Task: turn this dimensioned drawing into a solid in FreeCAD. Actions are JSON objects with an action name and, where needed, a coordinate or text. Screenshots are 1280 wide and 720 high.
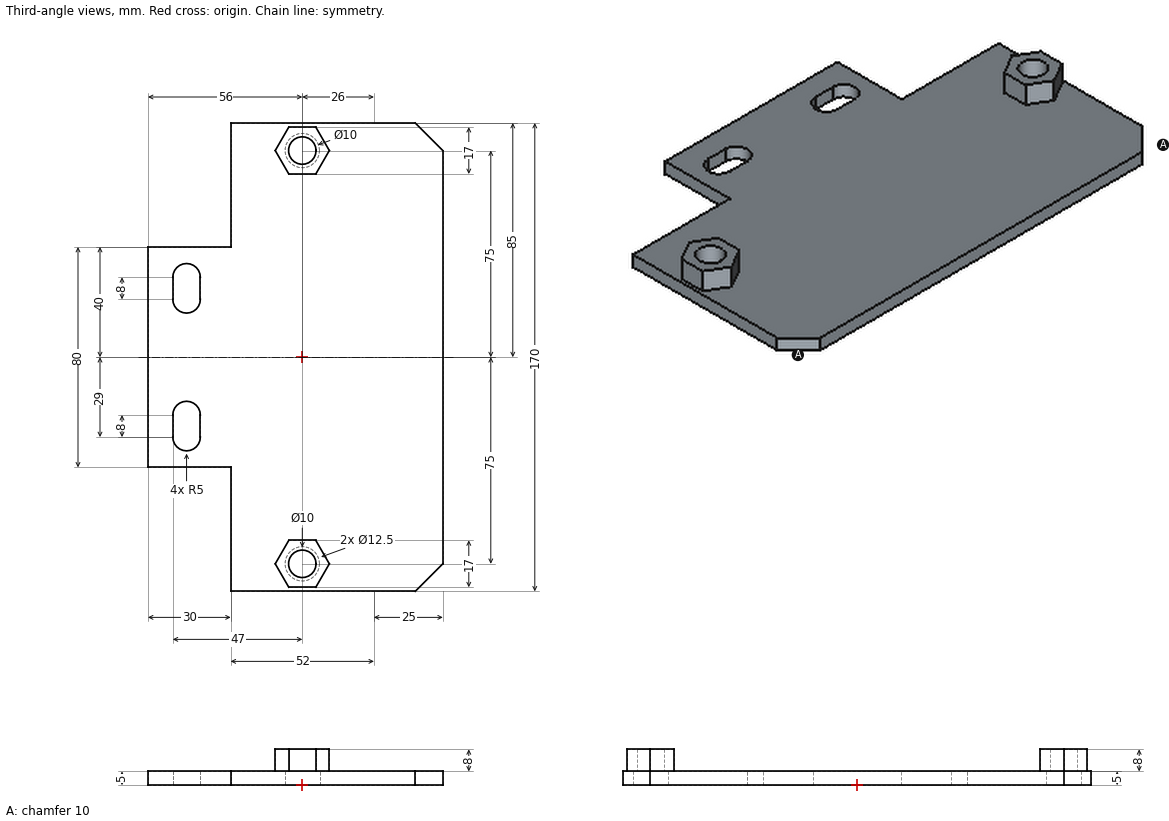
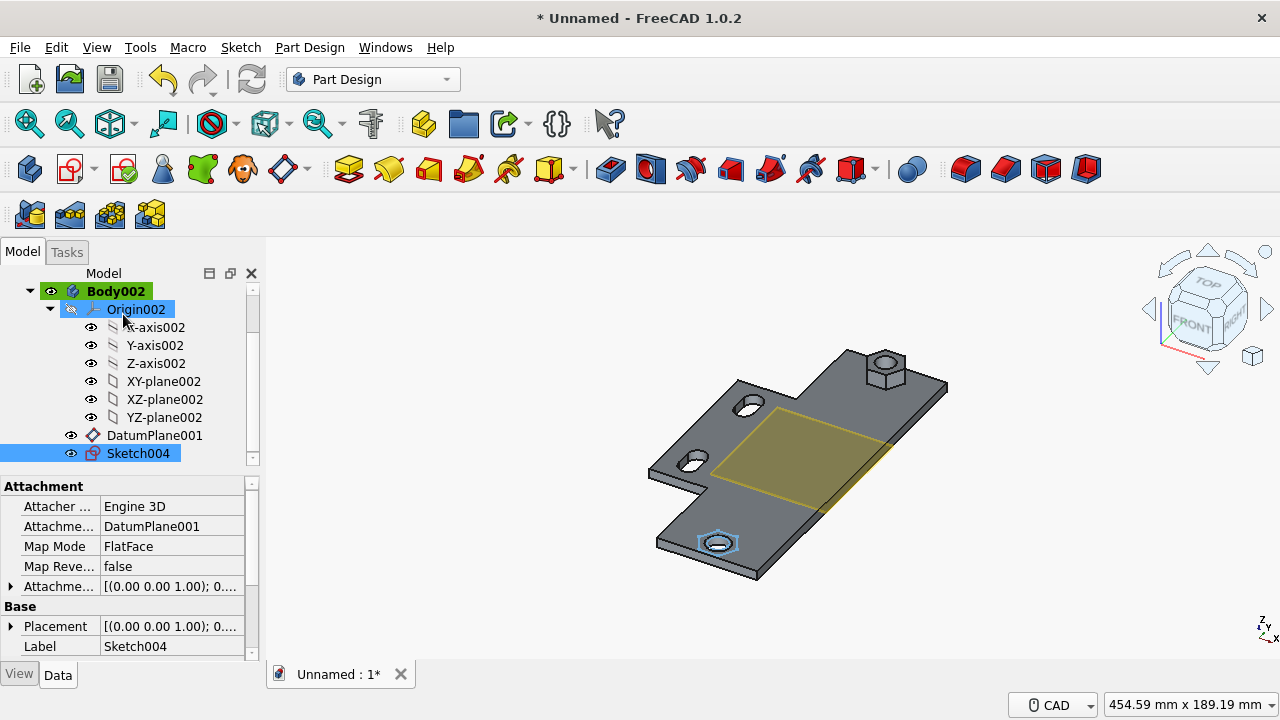
{"action": "left_click", "coordinate": [350, 170]}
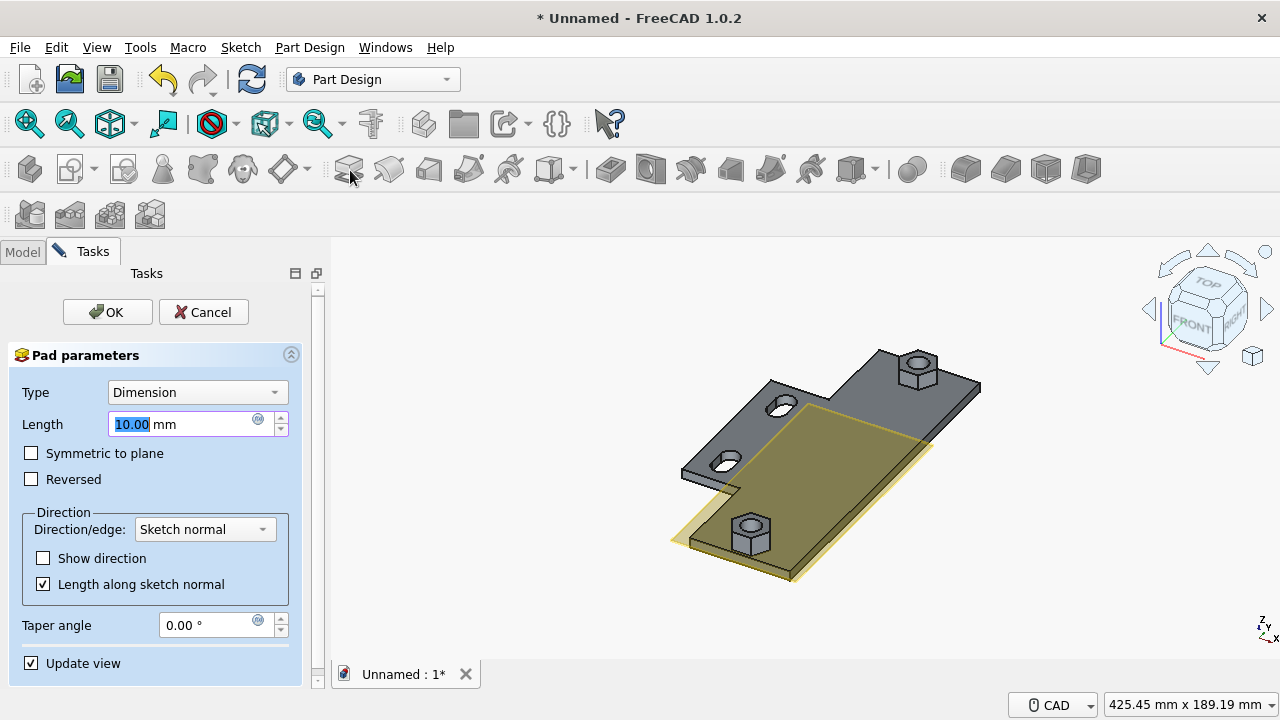
{"action": "type", "text": "8"}
{"action": "key", "text": "Tab"}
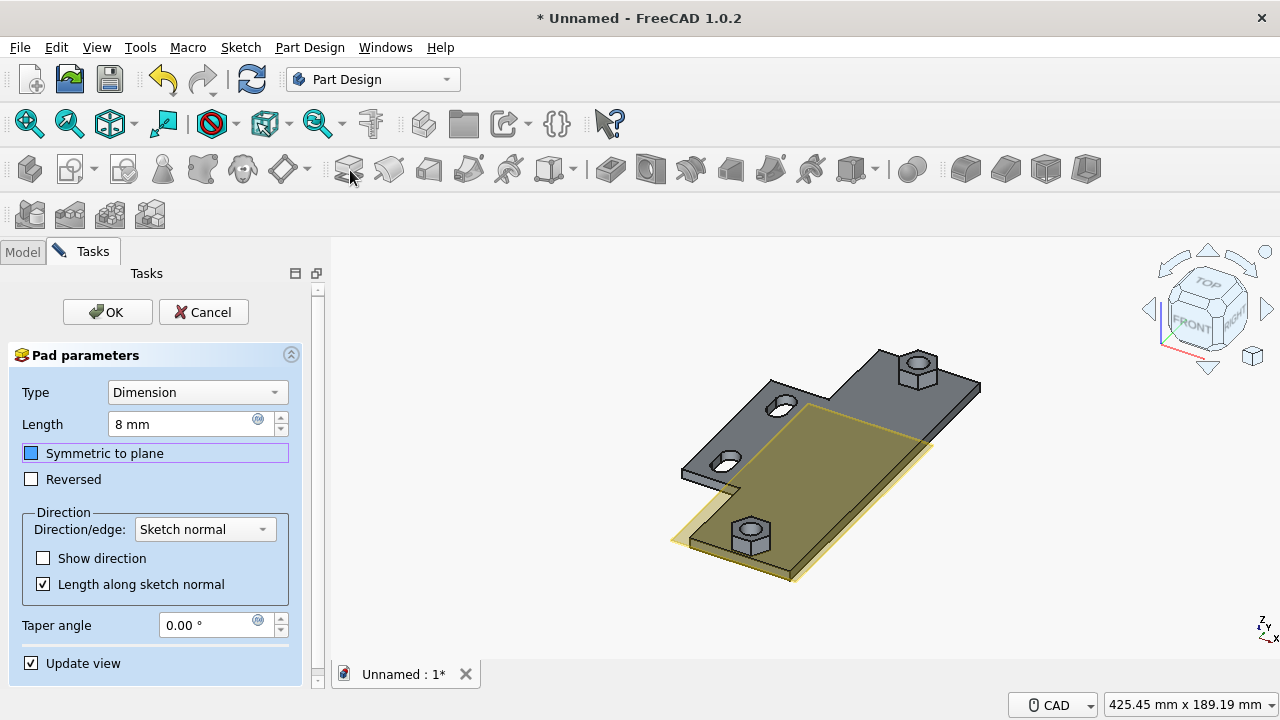
{"action": "left_click", "coordinate": [108, 312]}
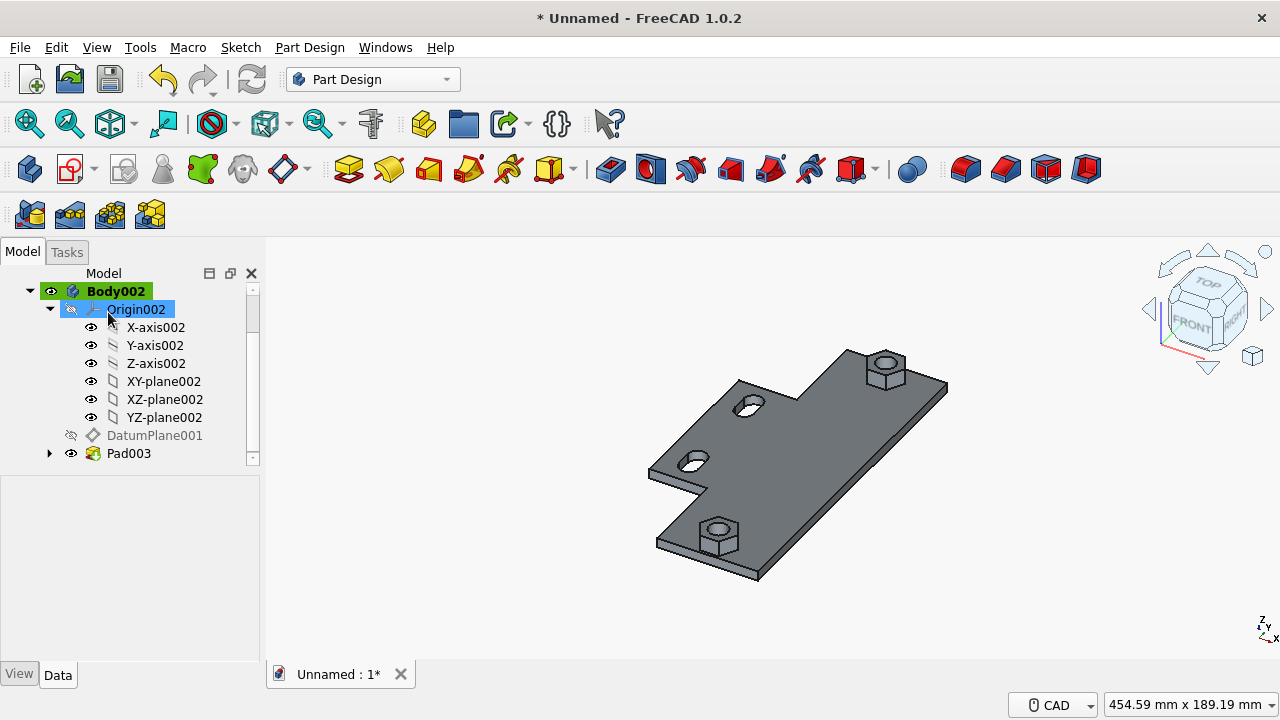
{"action": "left_click", "coordinate": [30, 124]}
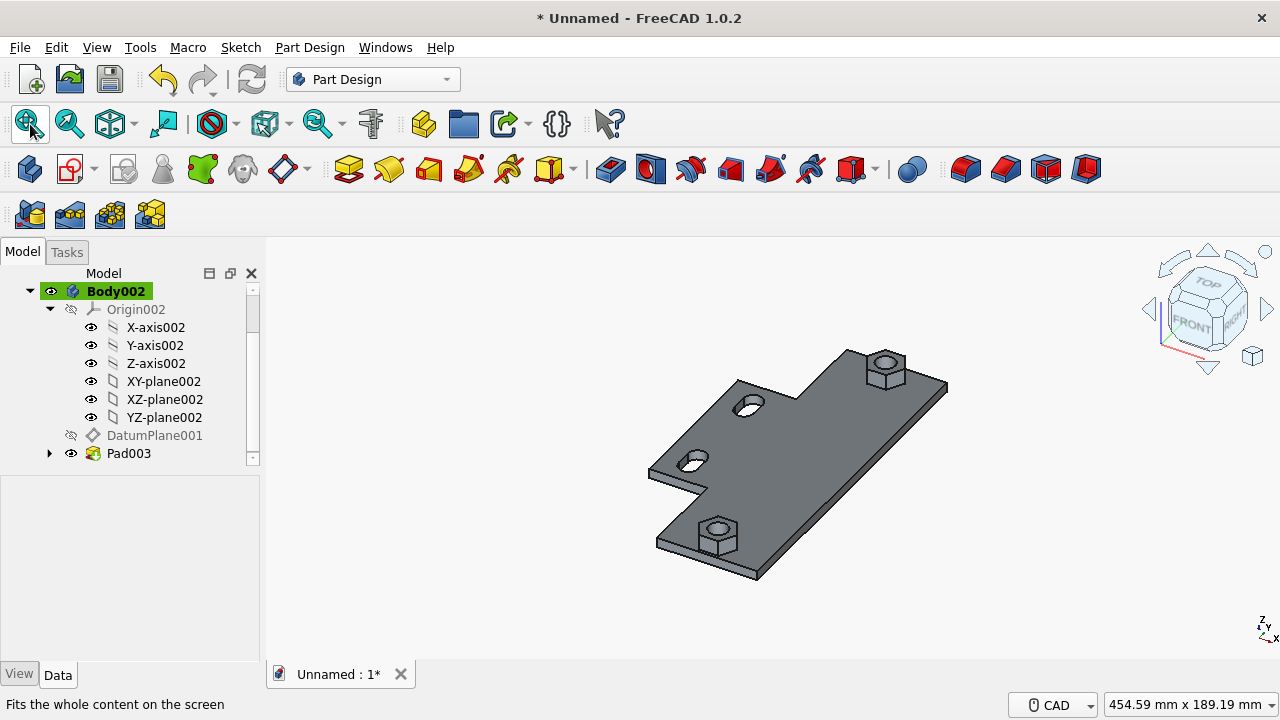
{"action": "left_click", "coordinate": [30, 170]}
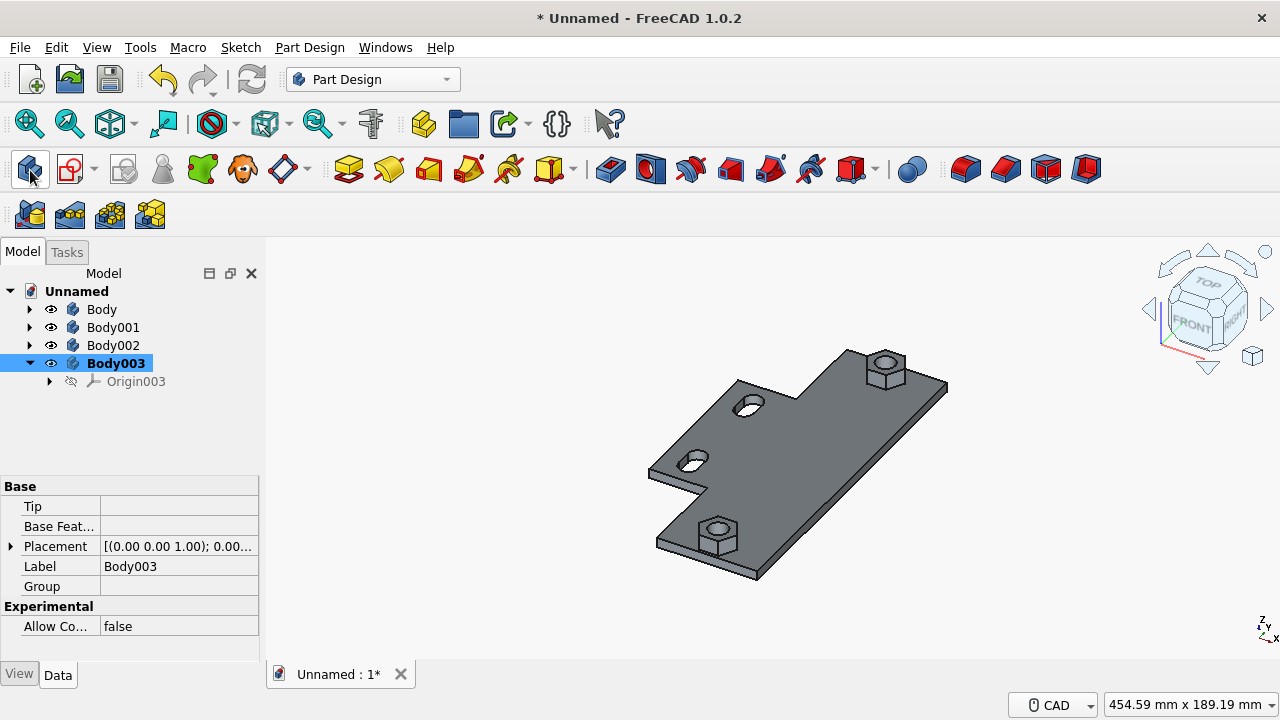
{"action": "left_click", "coordinate": [50, 381]}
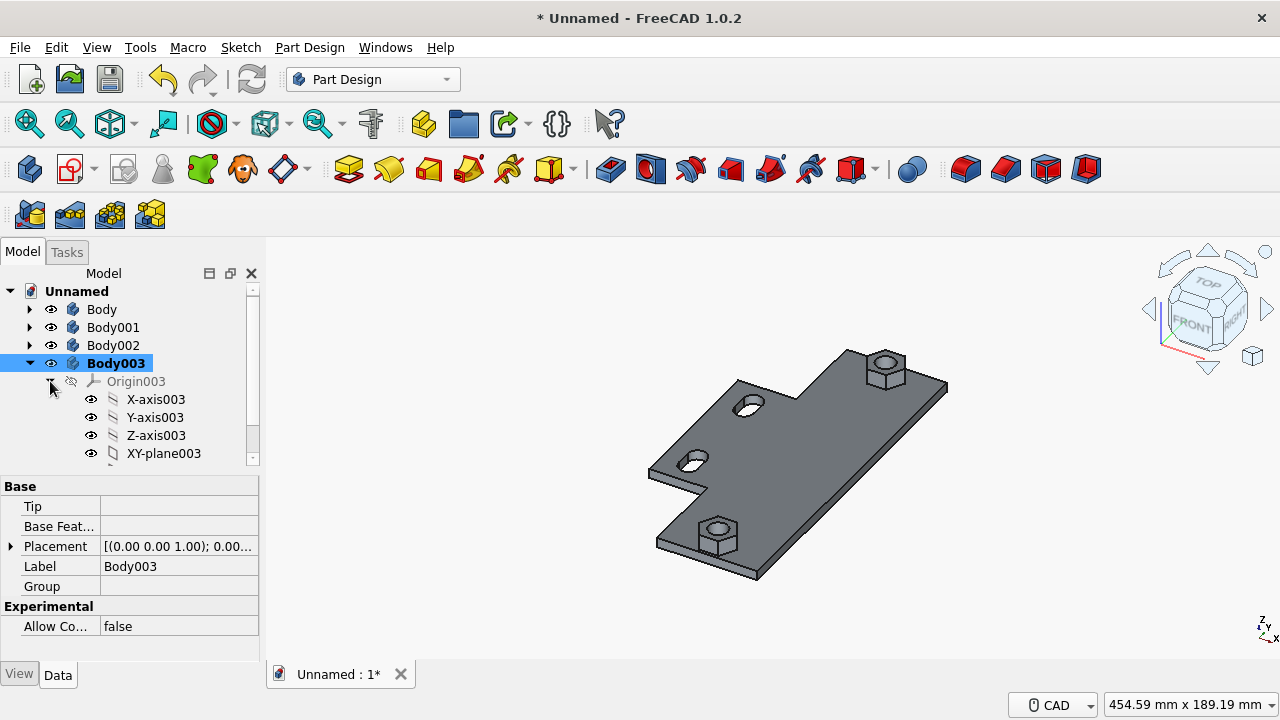
{"action": "left_click", "coordinate": [136, 453]}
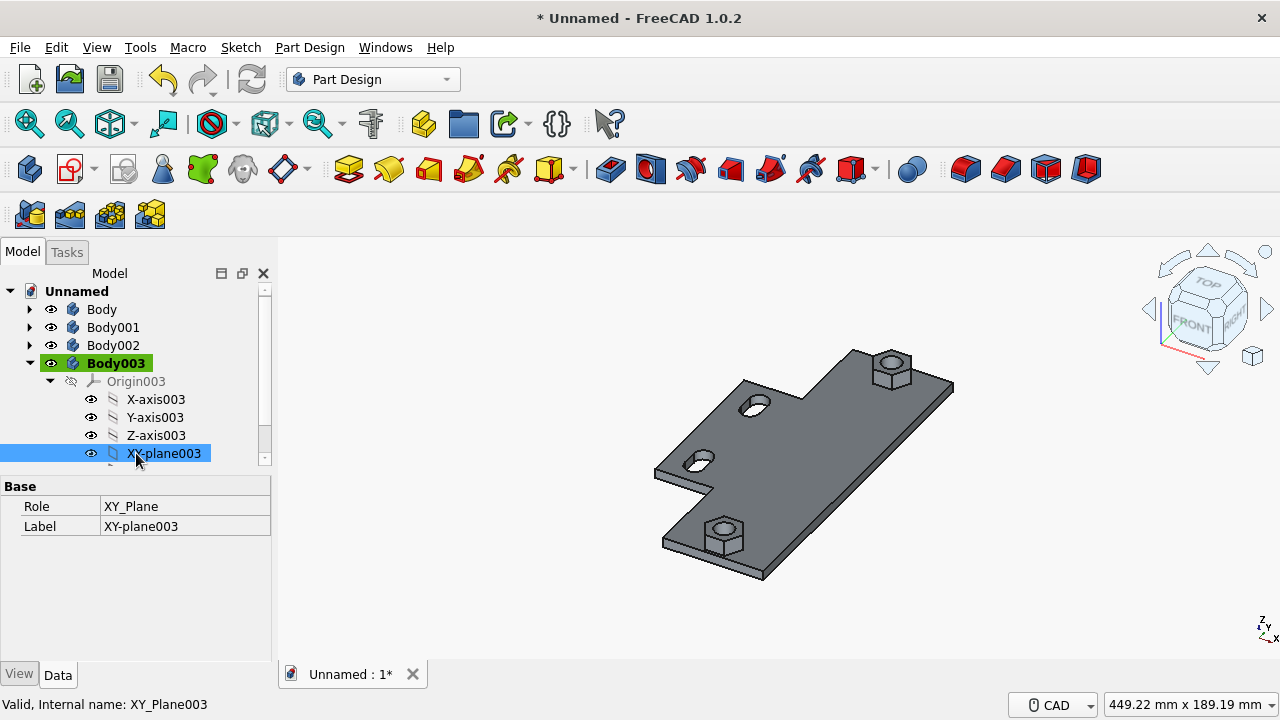
{"action": "left_click", "coordinate": [284, 170]}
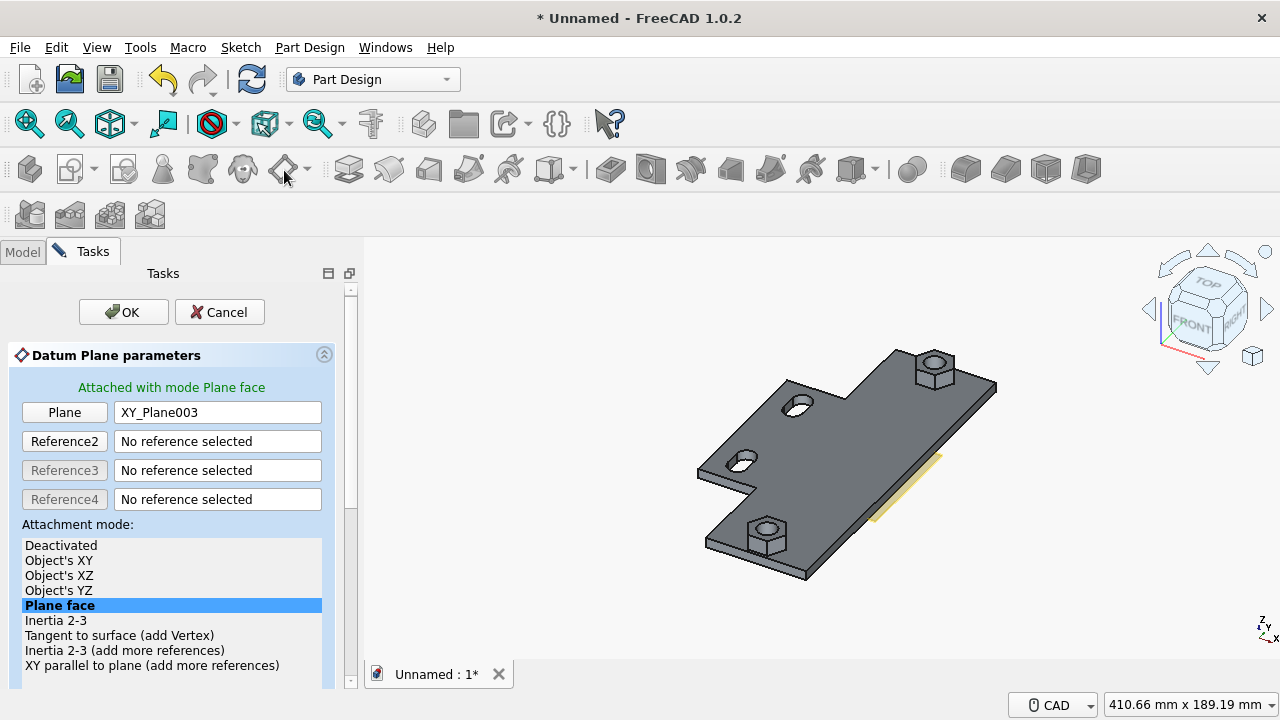
{"action": "scroll", "coordinate": [351, 486], "scroll_direction": "down", "scroll_amount": 4}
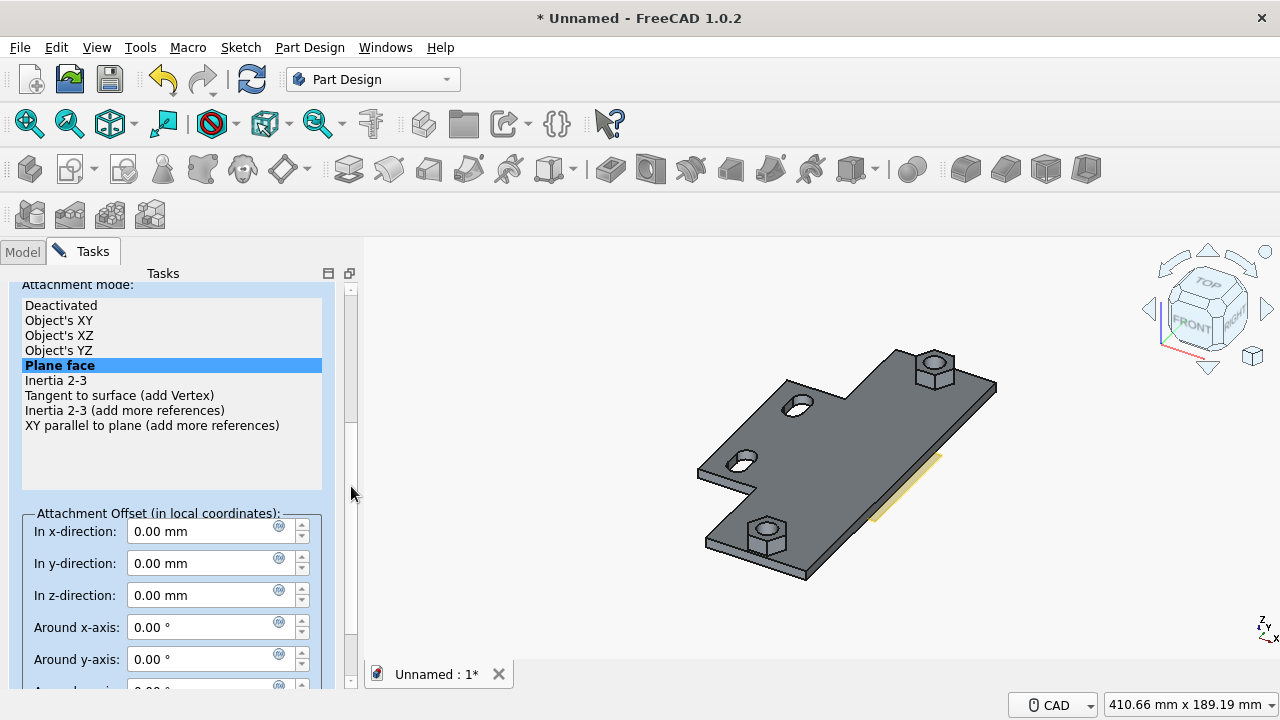
{"action": "triple_click", "coordinate": [210, 595]}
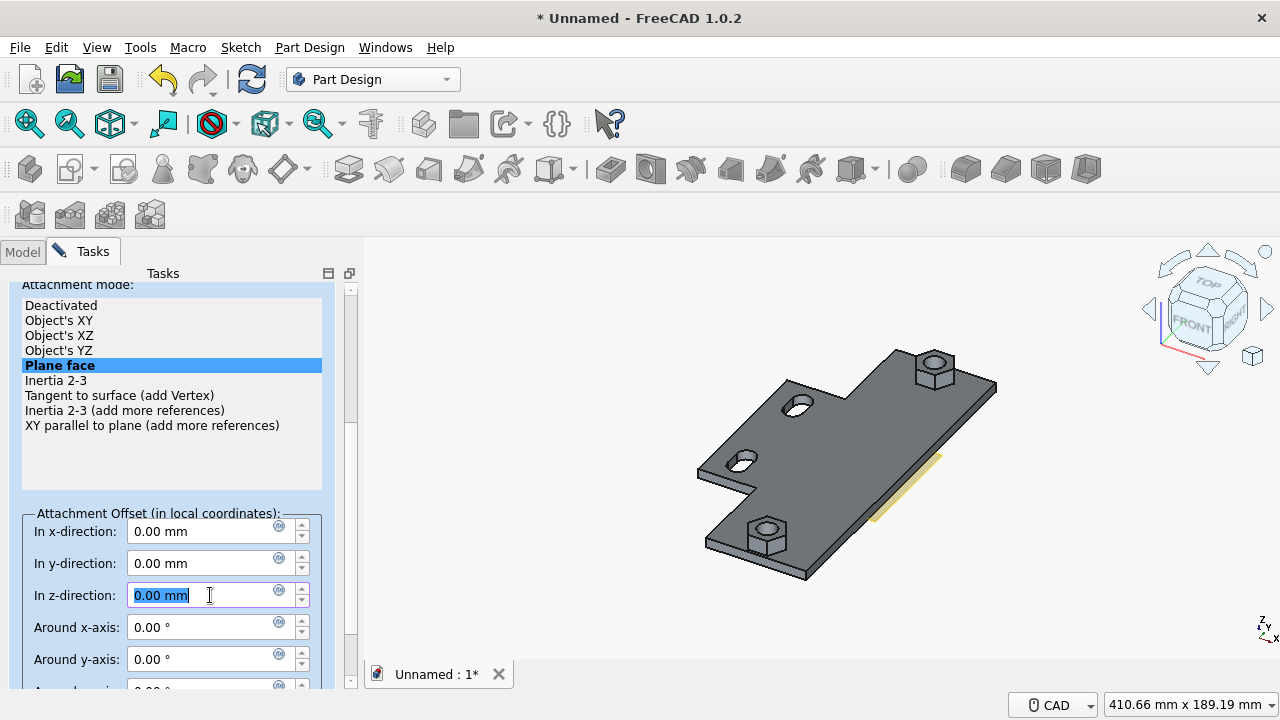
{"action": "type", "text": "5"}
{"action": "key", "text": "Tab"}